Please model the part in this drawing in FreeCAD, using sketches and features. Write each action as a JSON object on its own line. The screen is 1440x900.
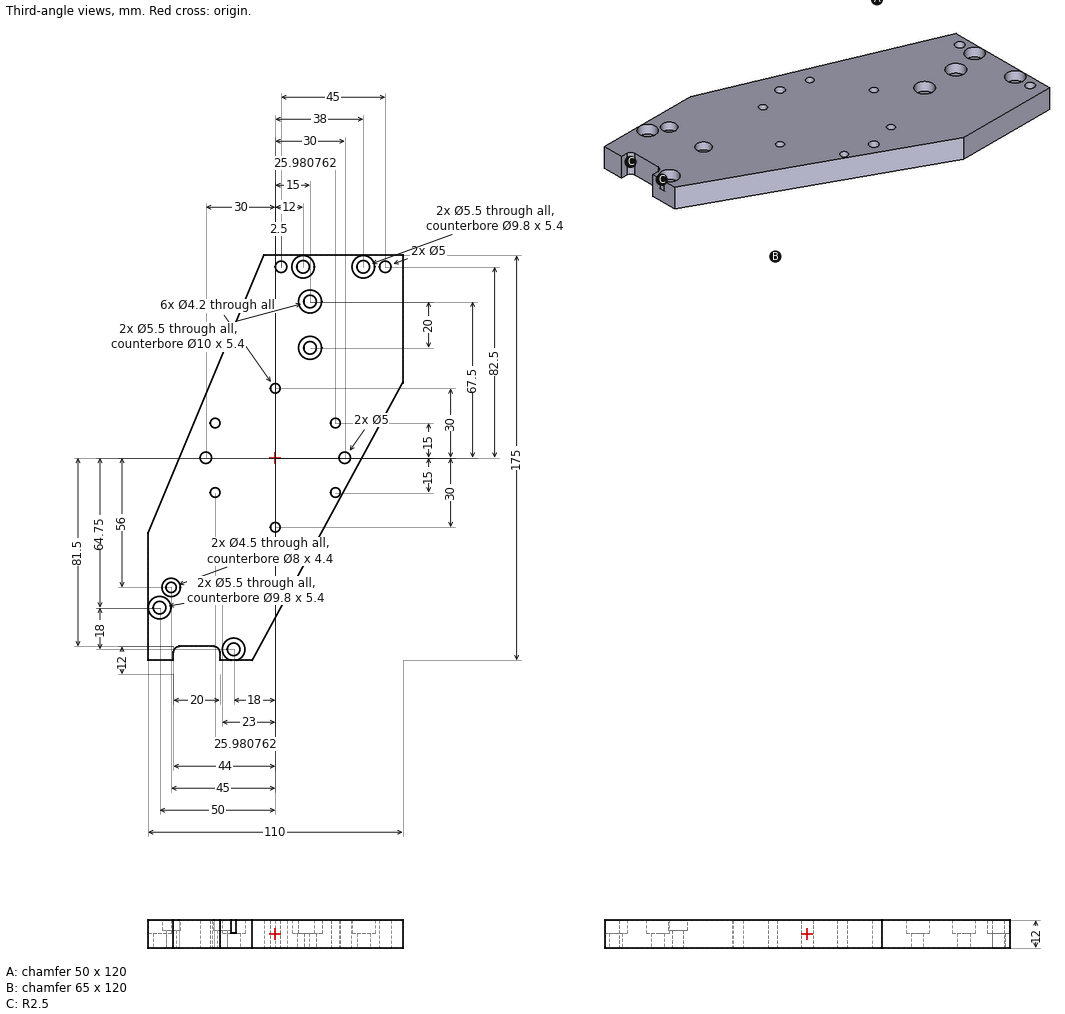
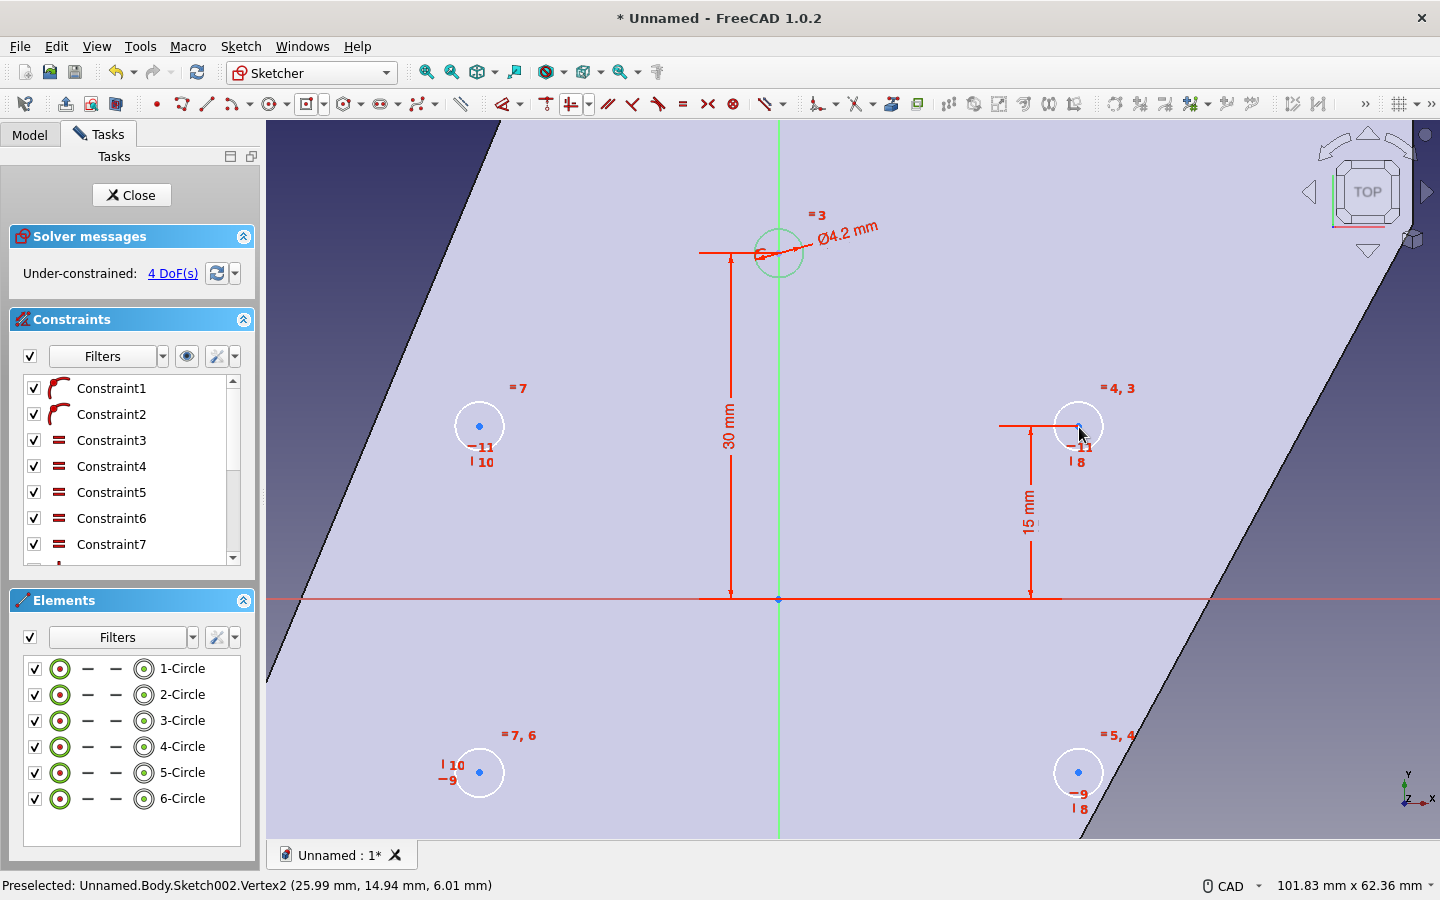
{"action": "left_click", "coordinate": [1079, 773]}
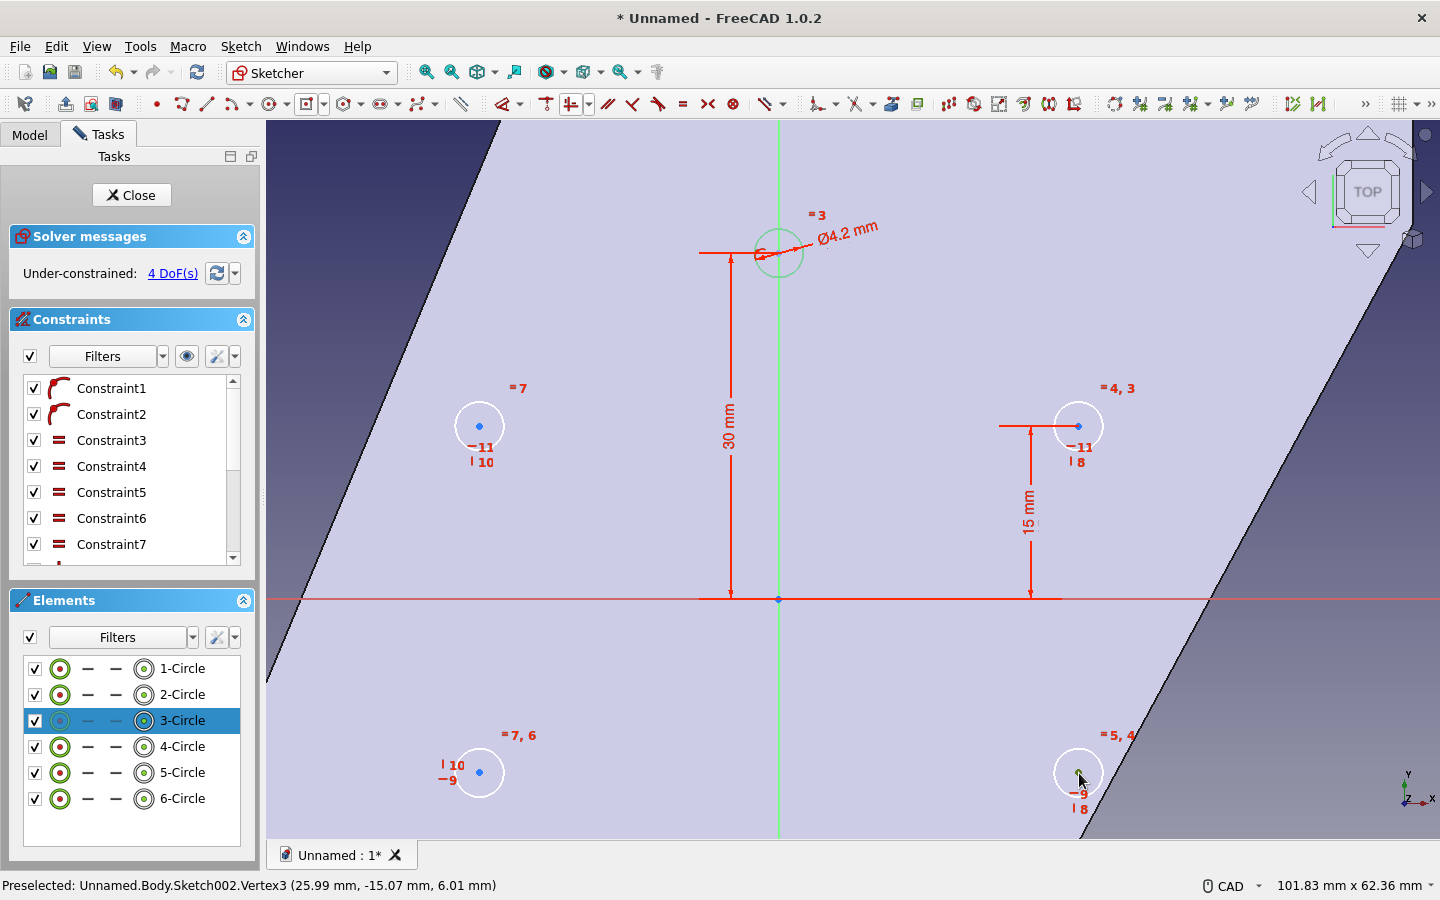
{"action": "key", "text": "i"}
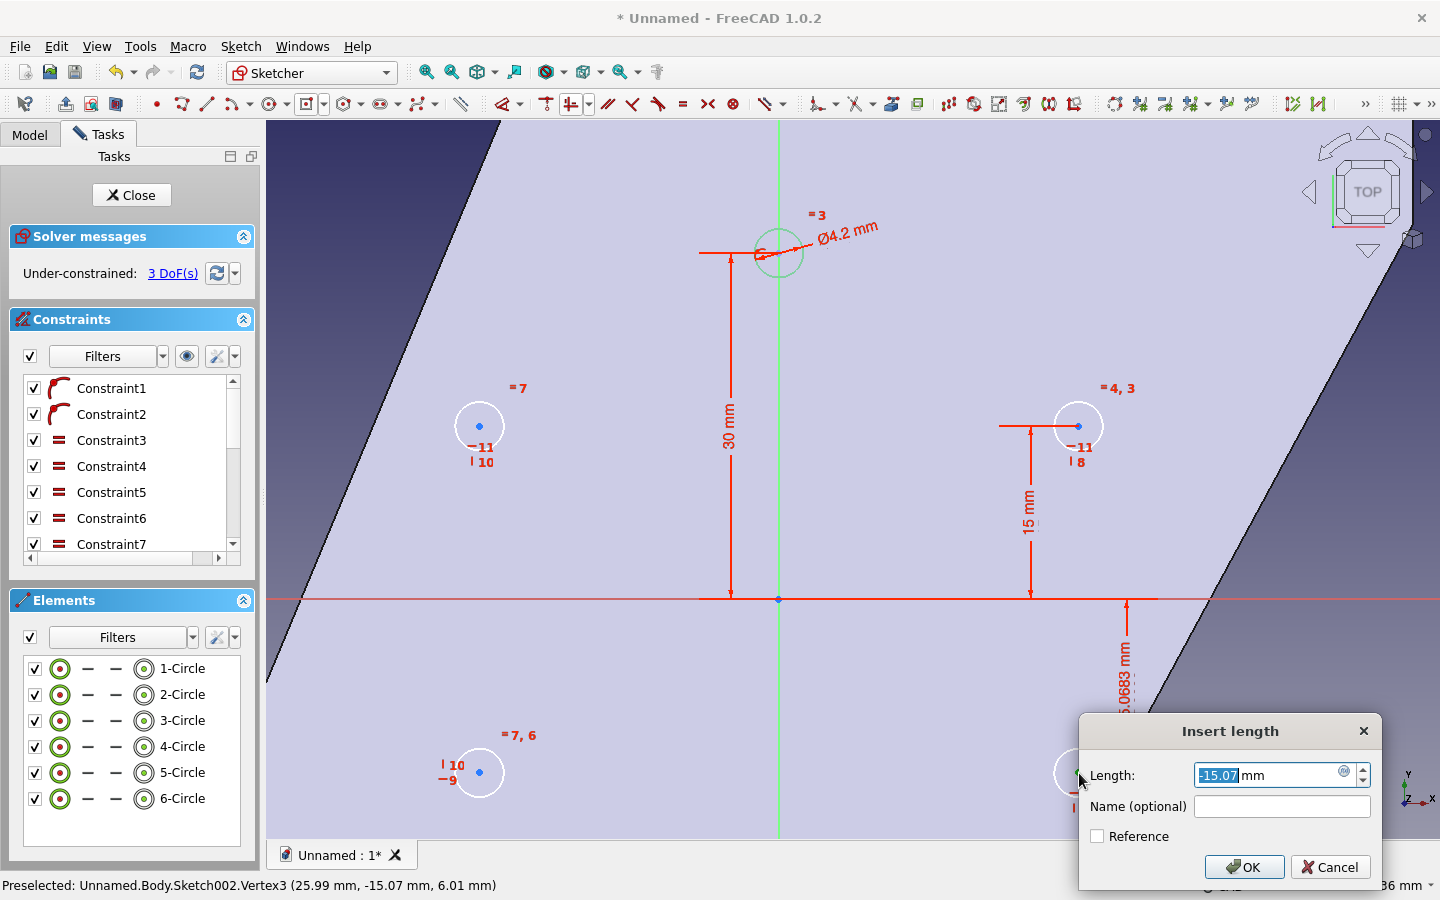
{"action": "type", "text": "-15"}
{"action": "key", "text": "Return"}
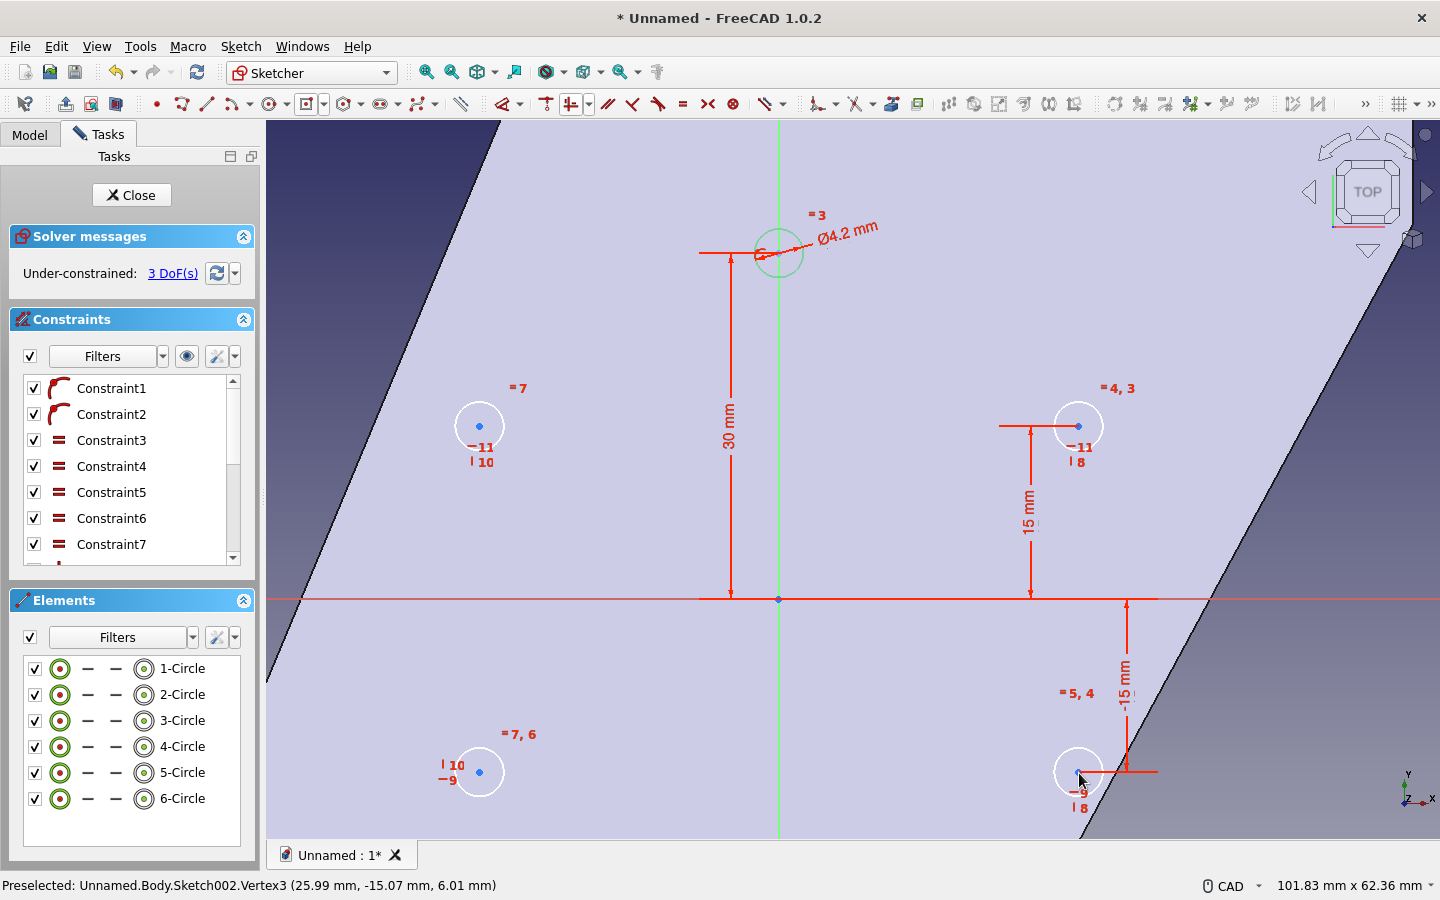
{"action": "scroll", "coordinate": [796, 236], "scroll_direction": "down", "scroll_amount": 2}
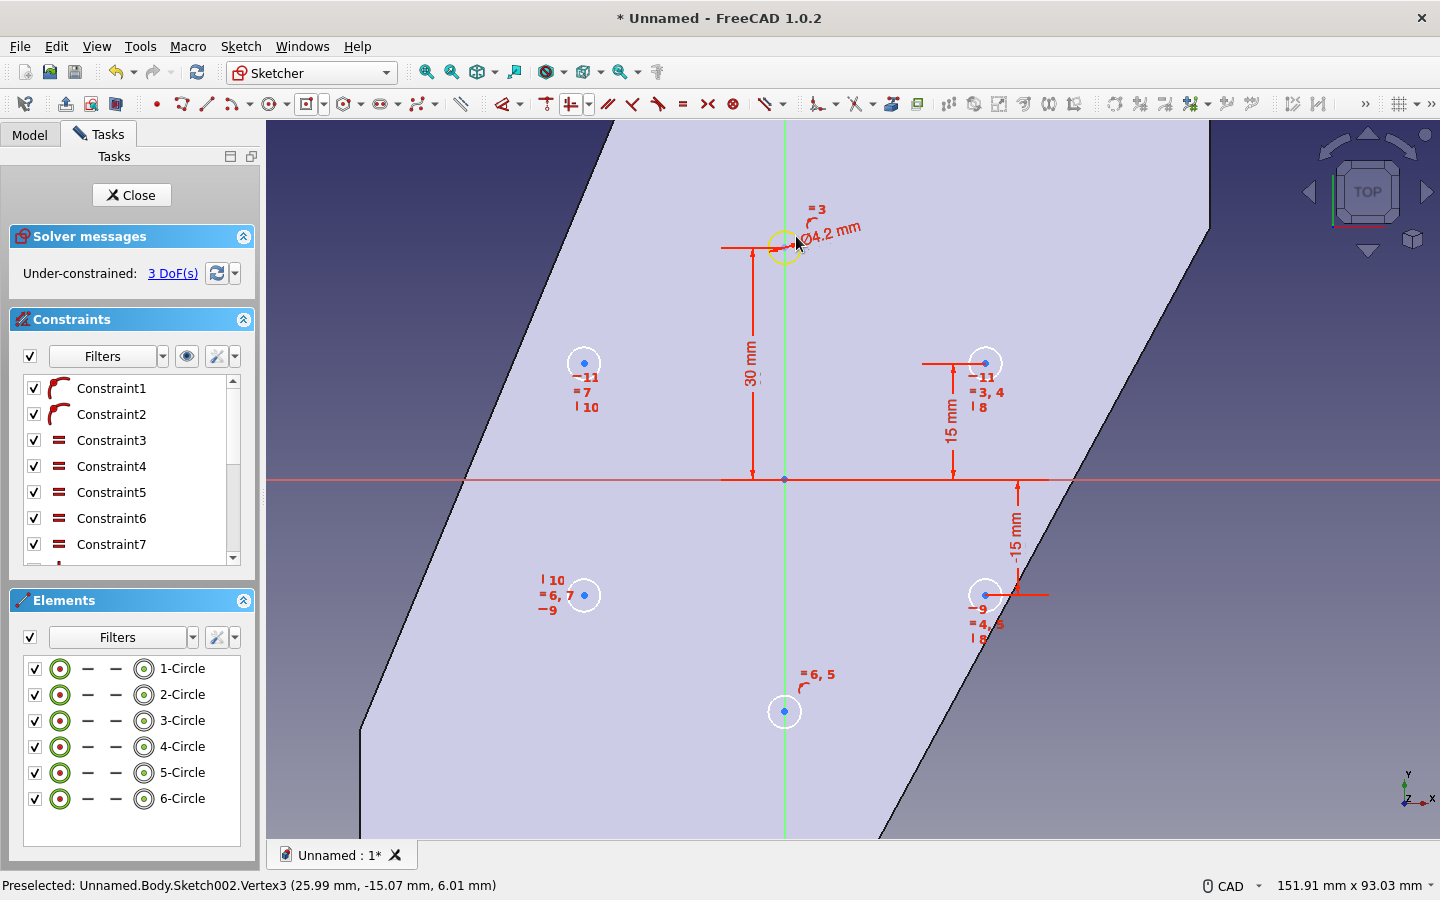
{"action": "left_click", "coordinate": [785, 712]}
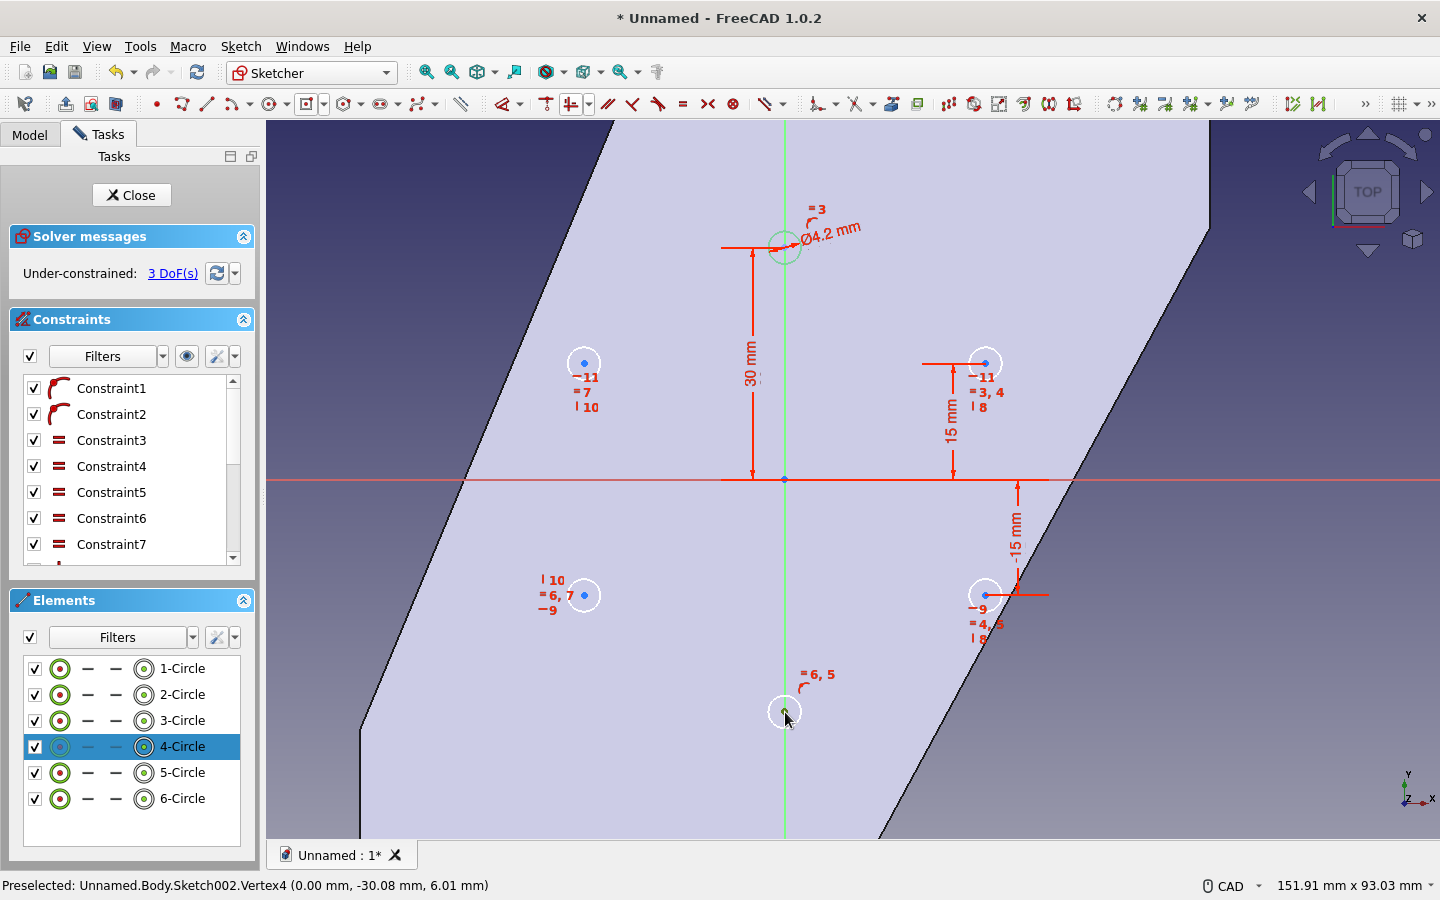
{"action": "key", "text": "i"}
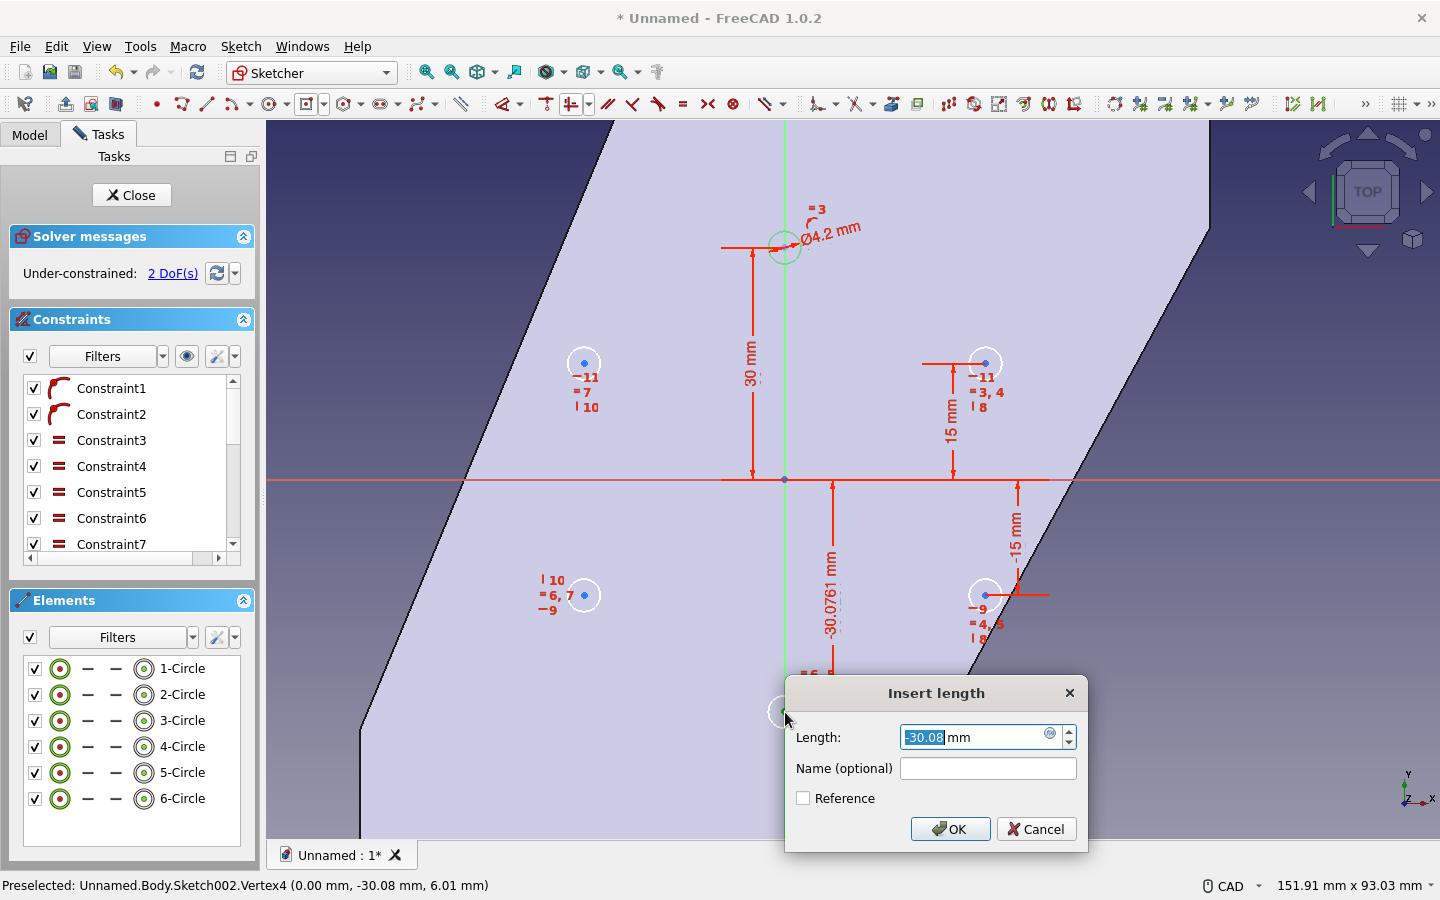
{"action": "type", "text": "-30"}
{"action": "key", "text": "Return"}